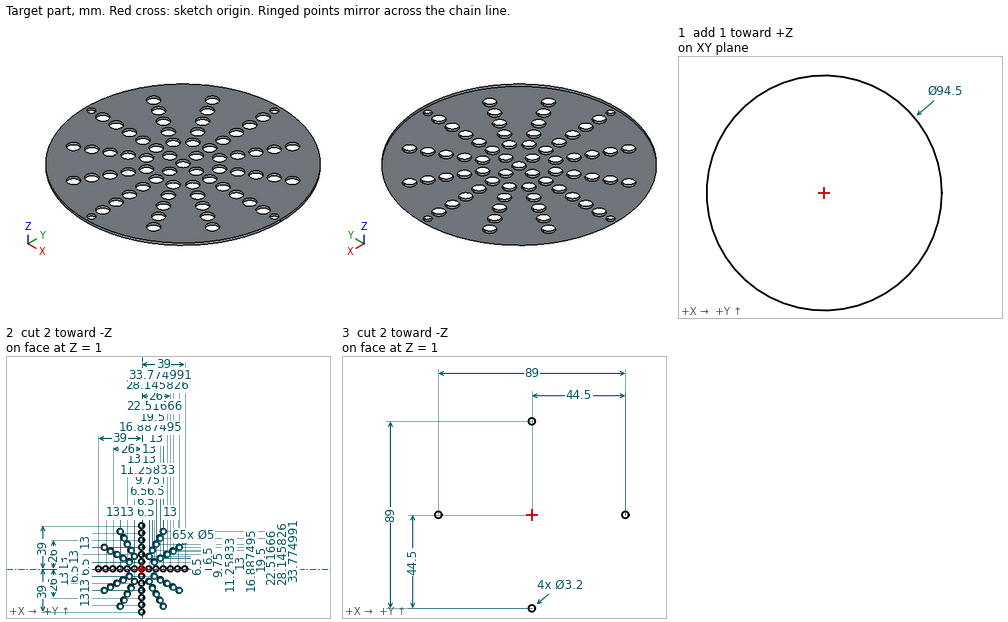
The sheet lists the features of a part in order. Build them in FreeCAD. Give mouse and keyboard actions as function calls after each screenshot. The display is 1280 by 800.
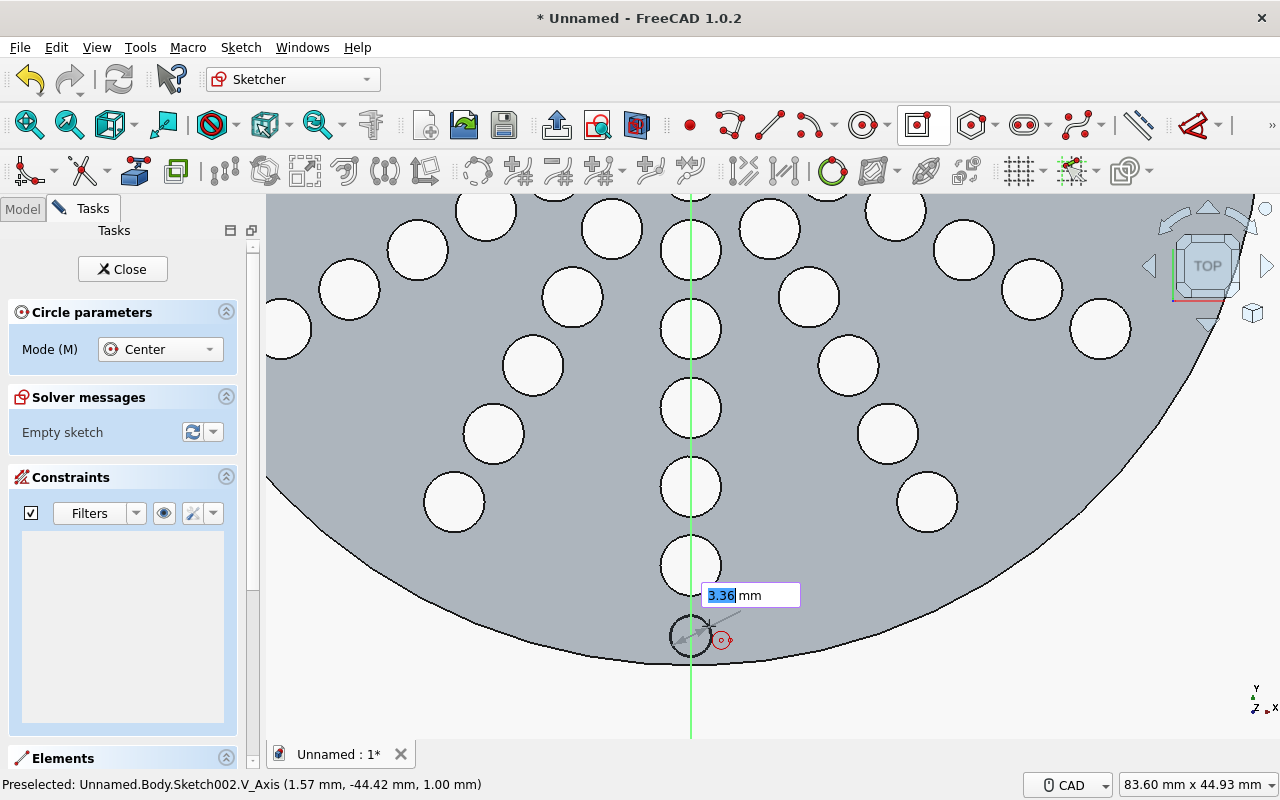
text(3.2)
key(Return)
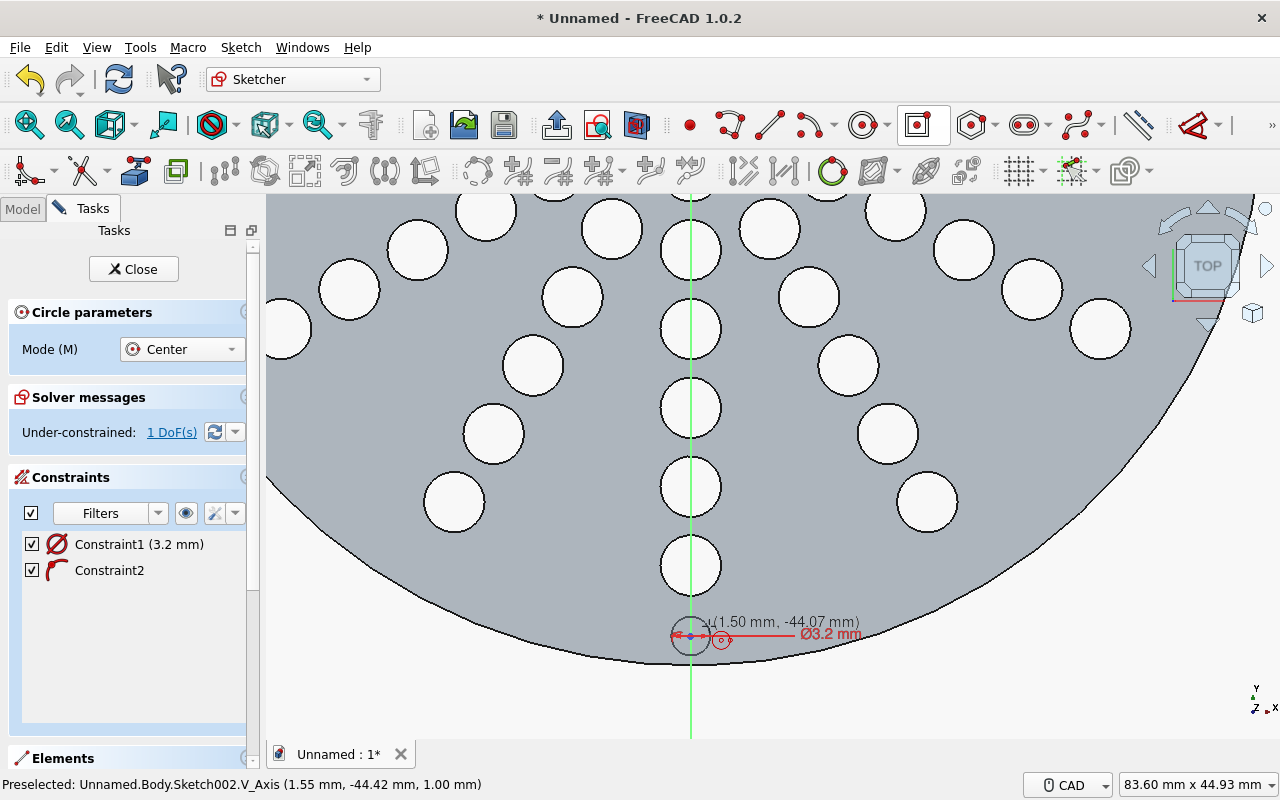
scroll(710, 628, down, 6)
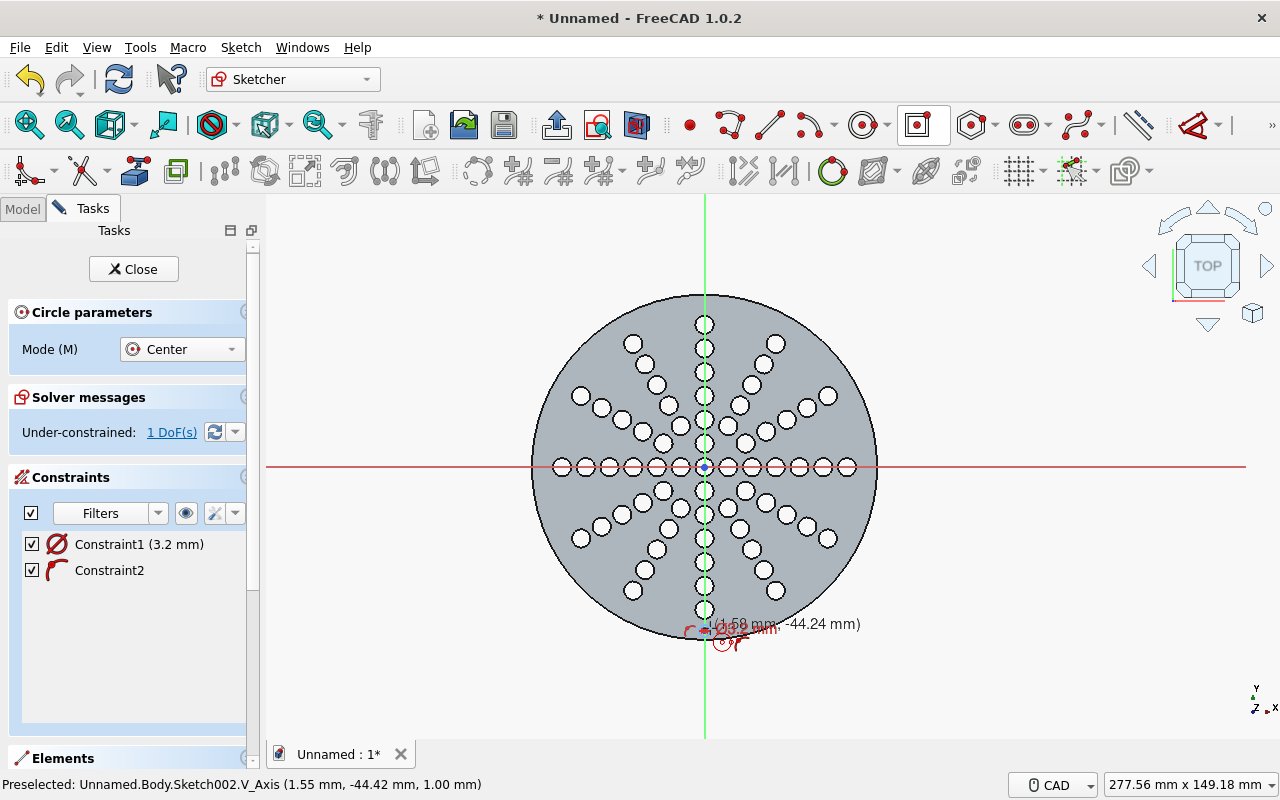
scroll(867, 467, up, 7)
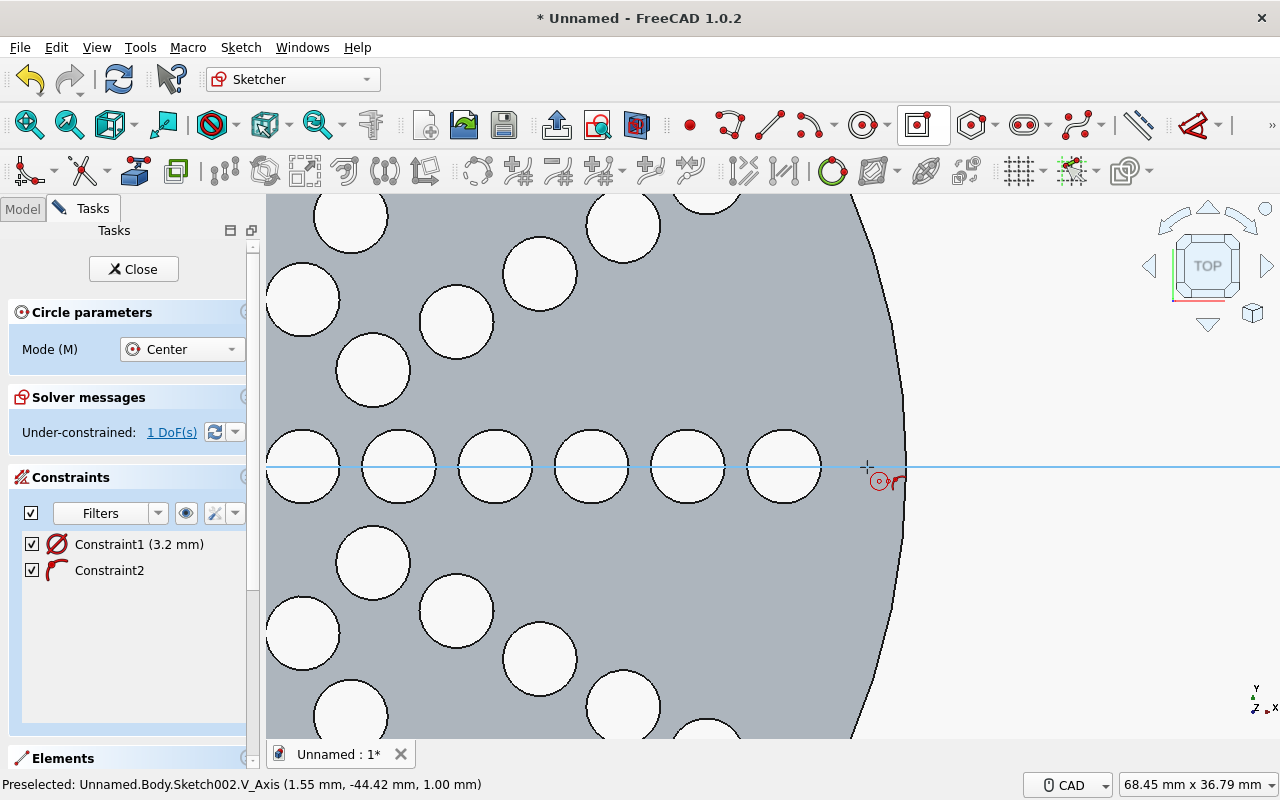
scroll(868, 466, down, 7)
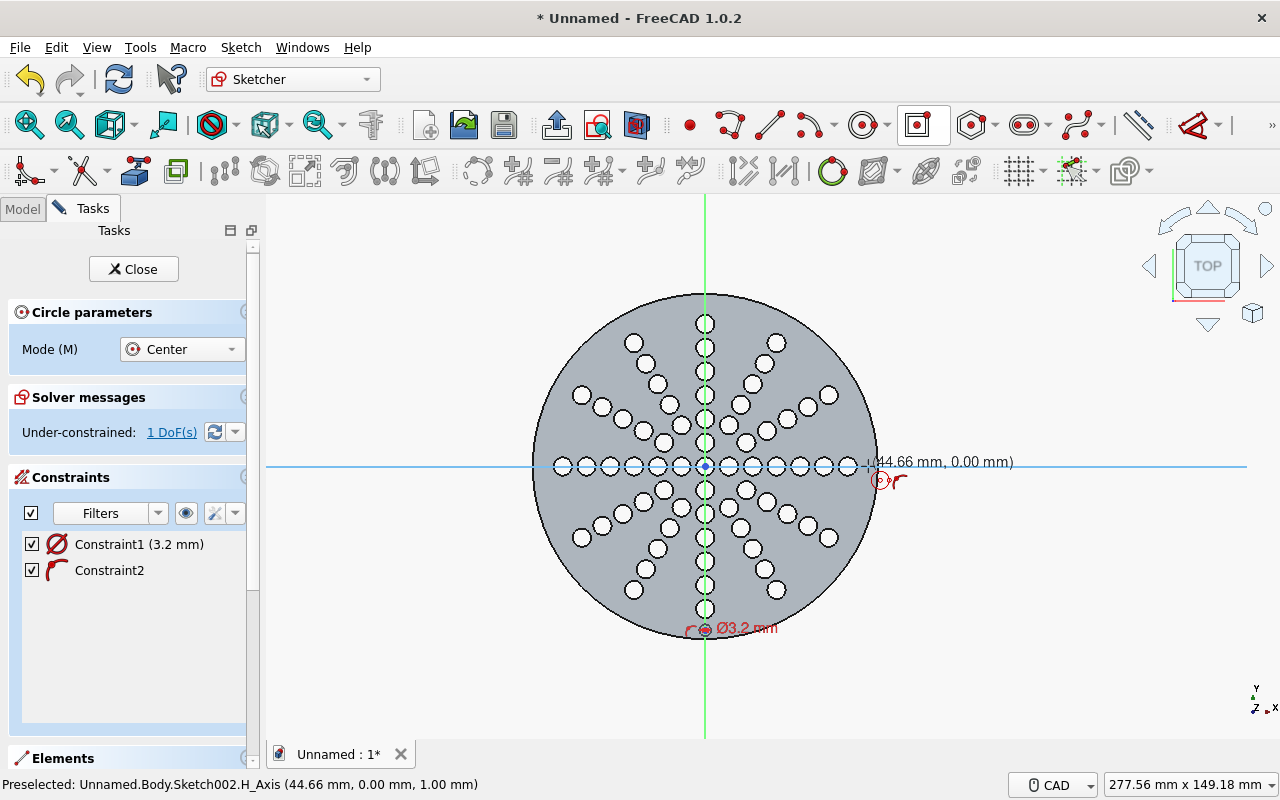
click(868, 467)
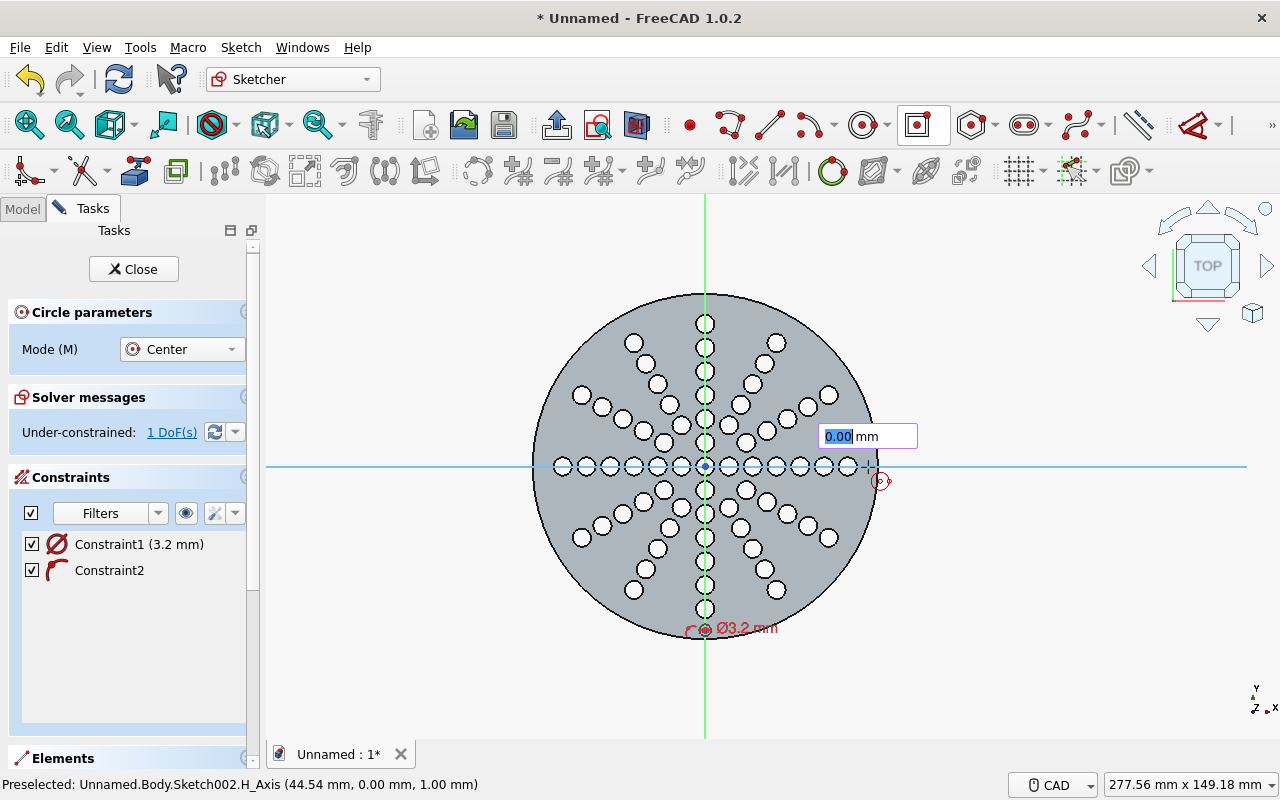
scroll(866, 472, up, 6)
move(864, 471)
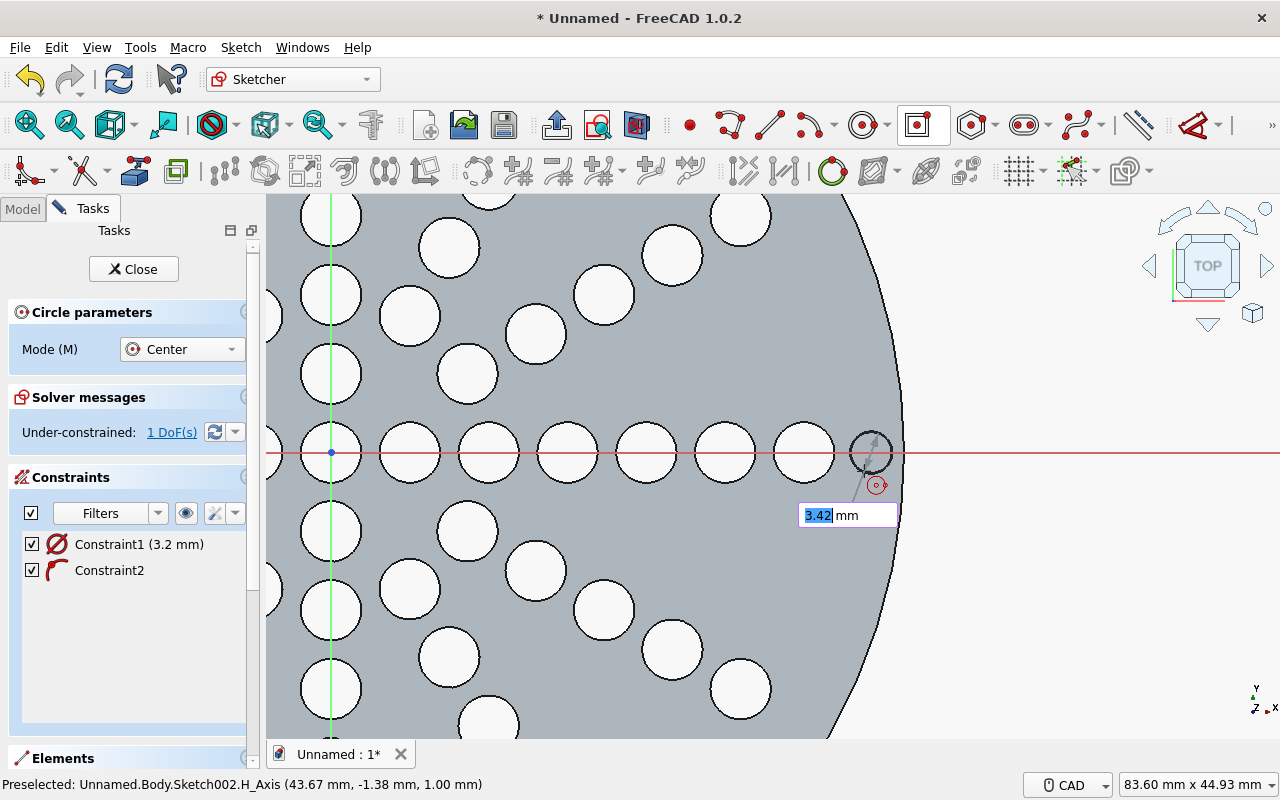
text(3.2)
key(Return)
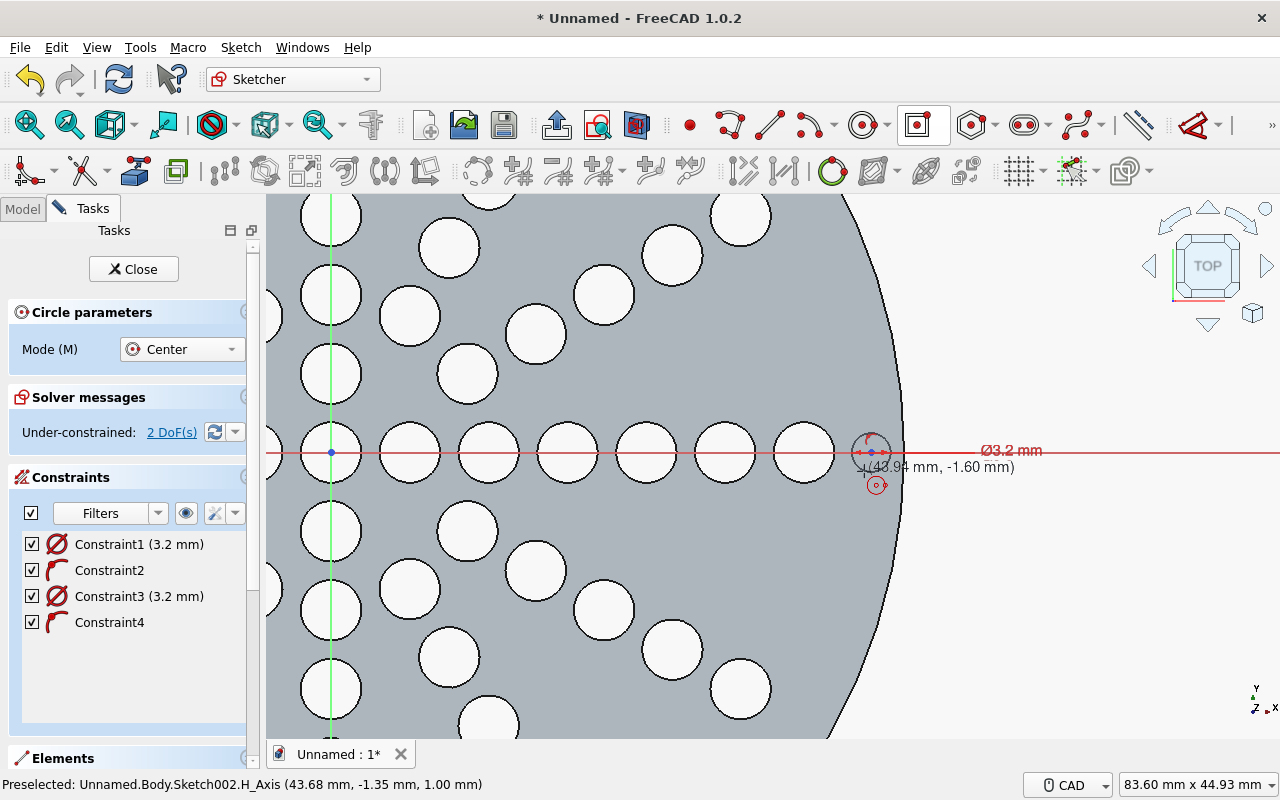
scroll(865, 473, down, 6)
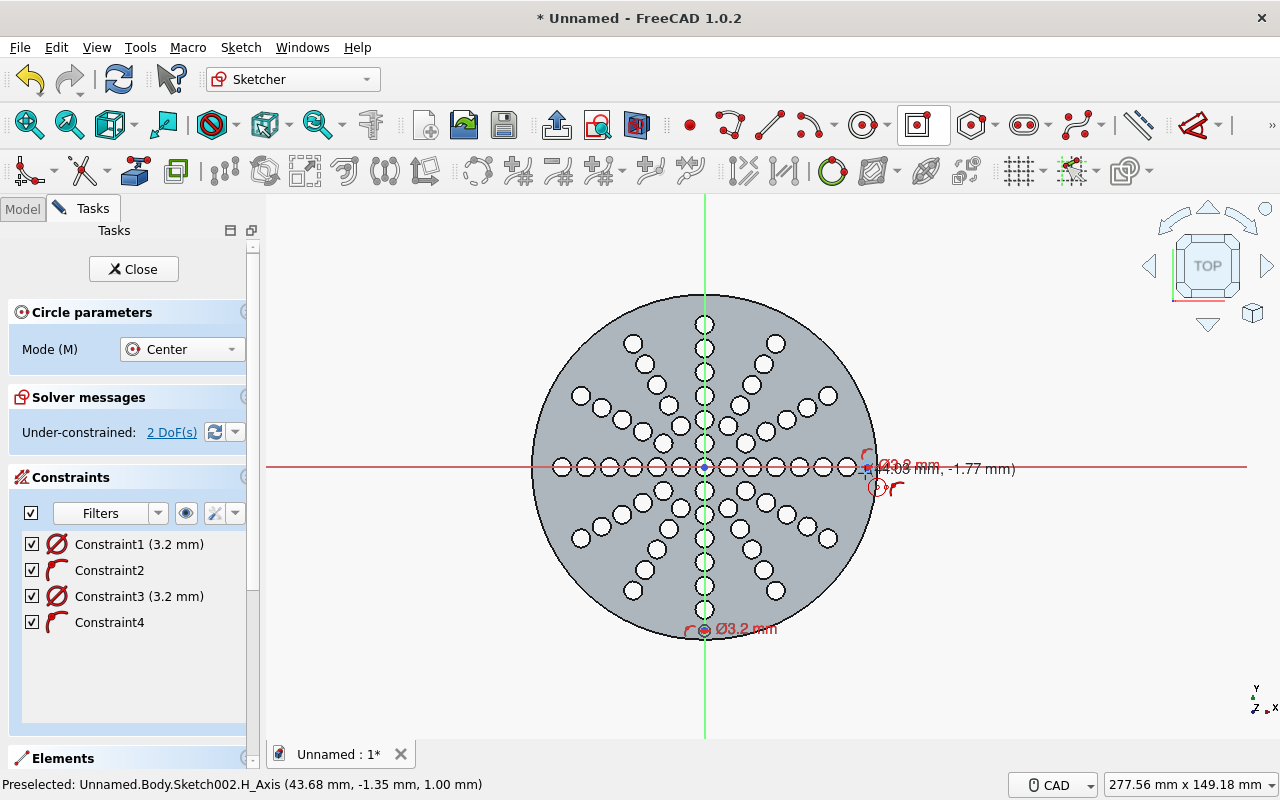
scroll(542, 467, up, 7)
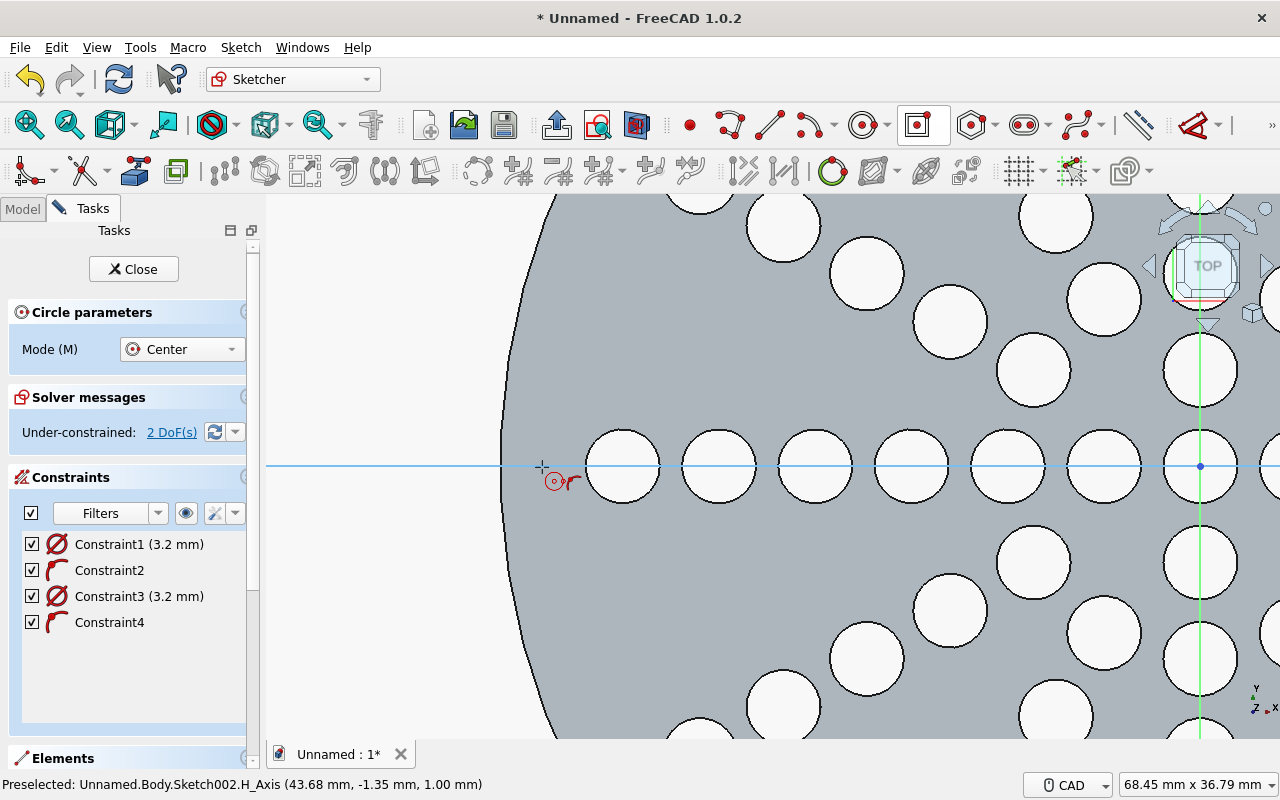
scroll(542, 467, down, 7)